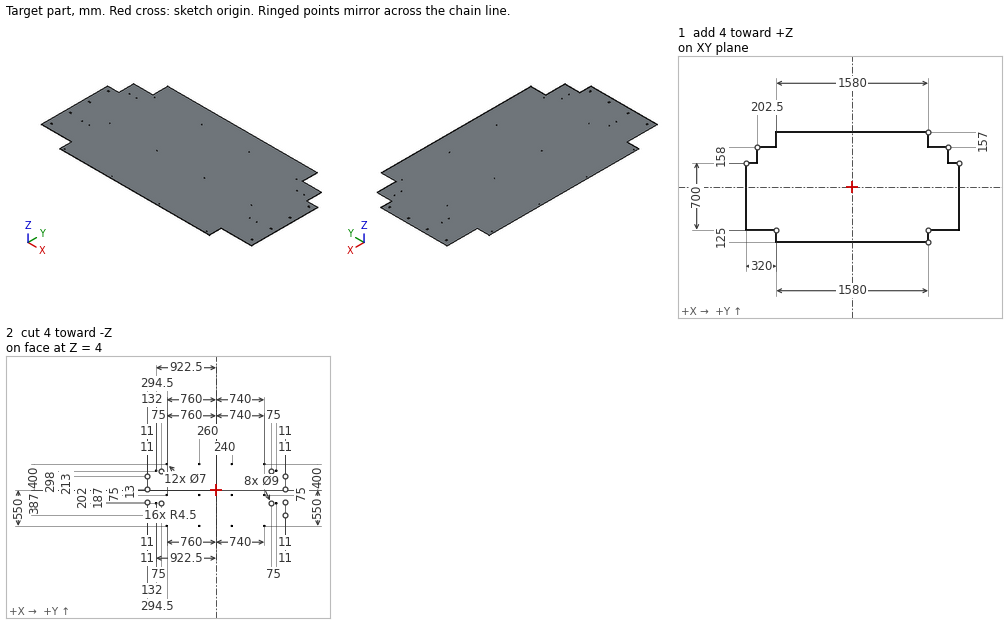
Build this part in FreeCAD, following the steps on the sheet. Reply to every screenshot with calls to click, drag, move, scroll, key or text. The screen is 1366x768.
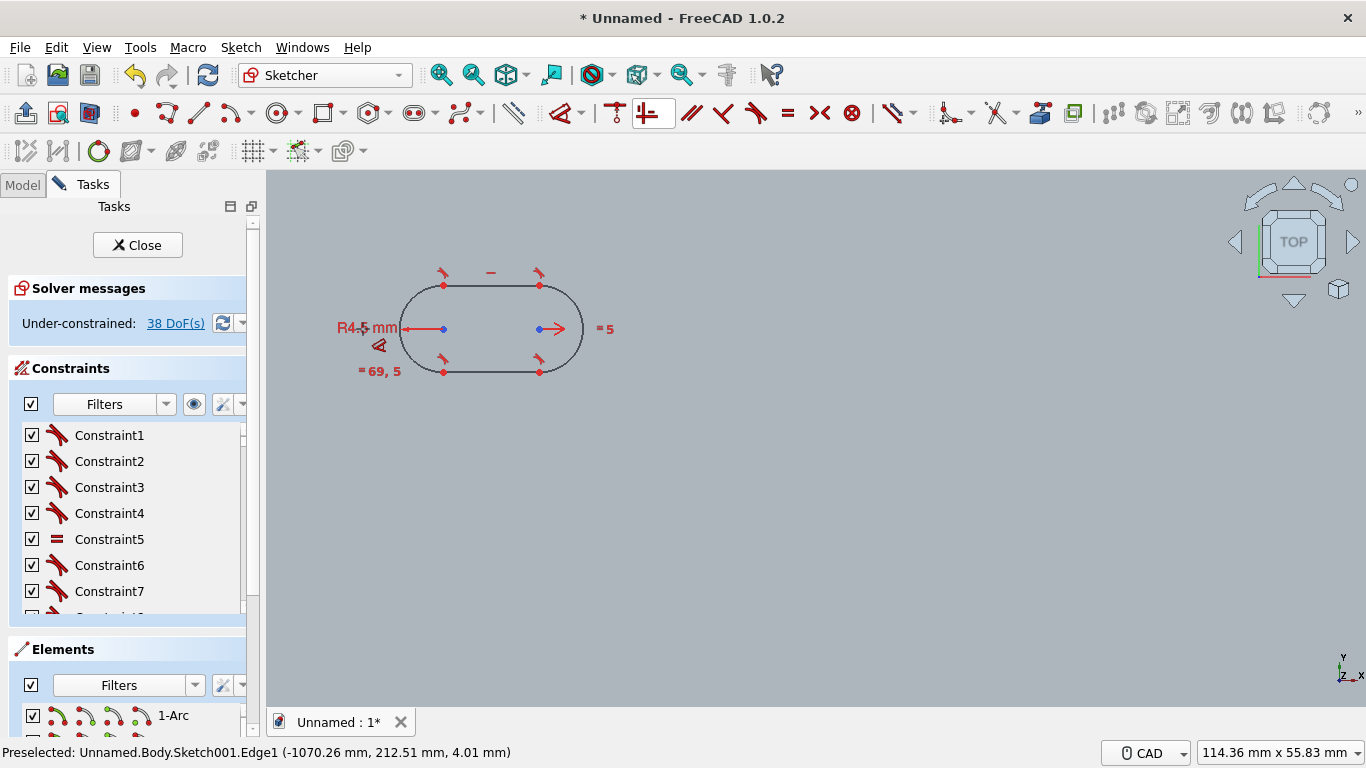
click(472, 286)
click(491, 252)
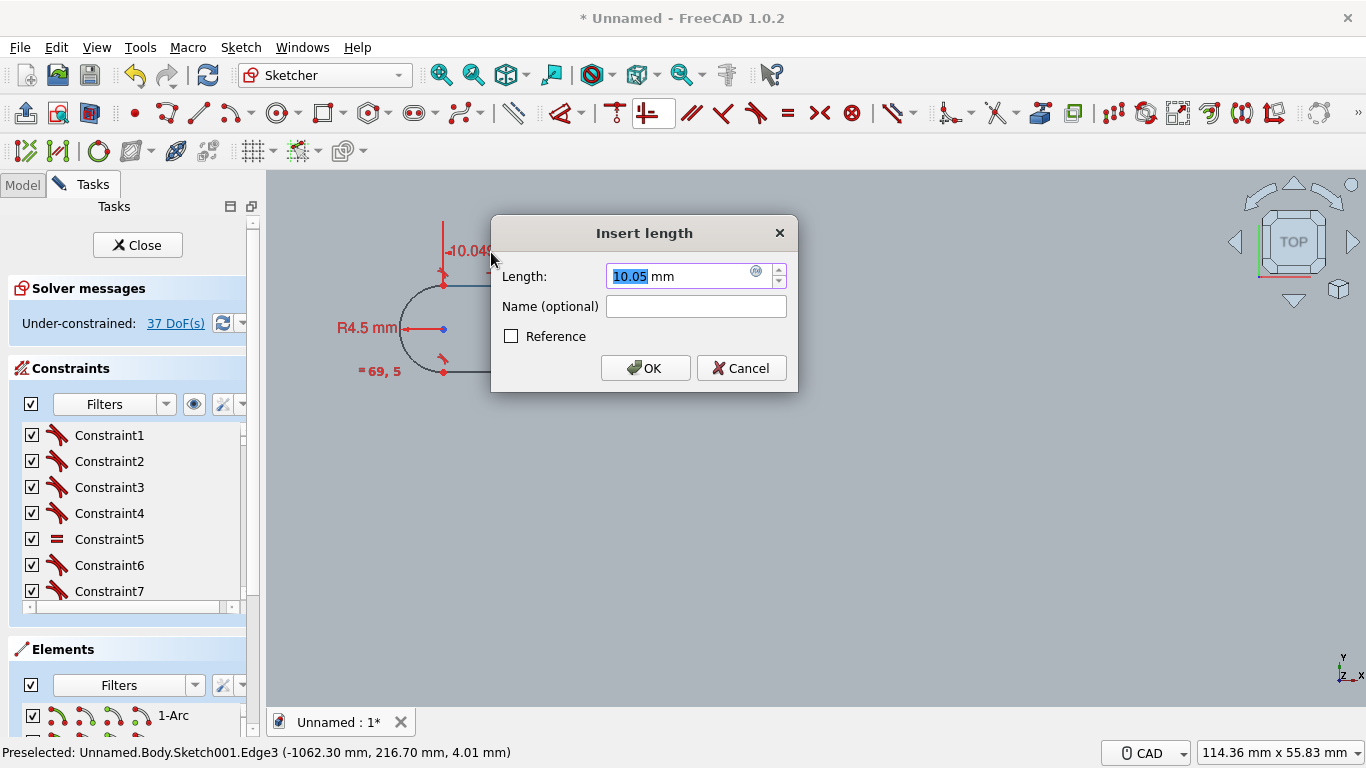
text(11)
key(Return)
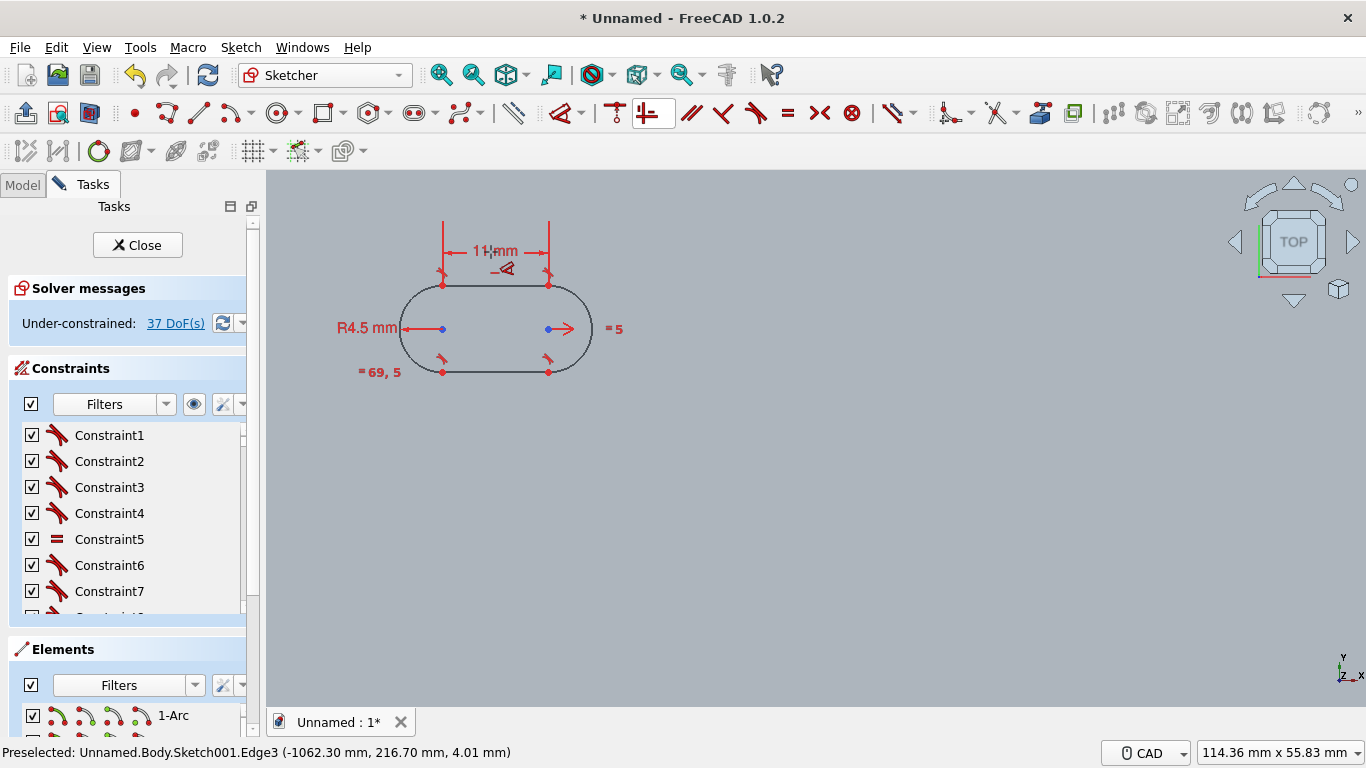
scroll(325, 326, down, 16)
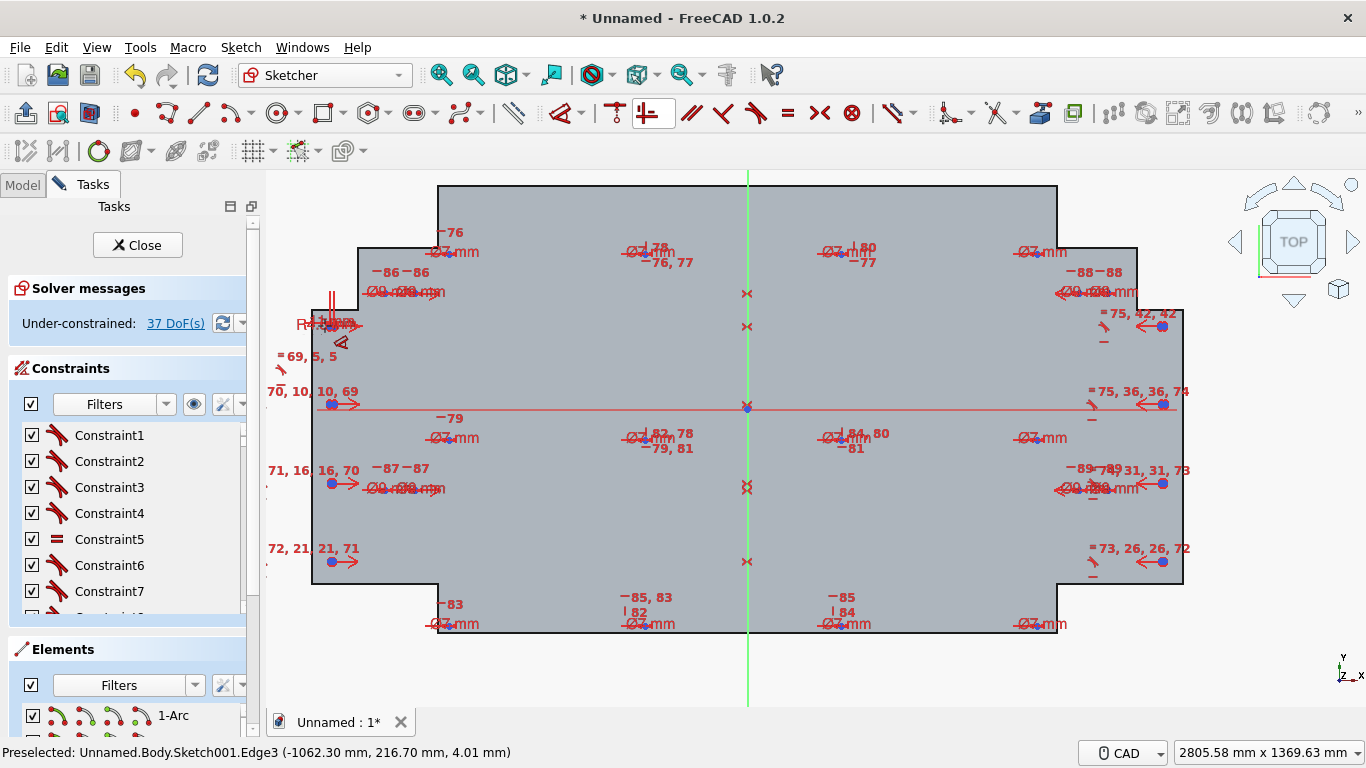
scroll(331, 403, up, 13)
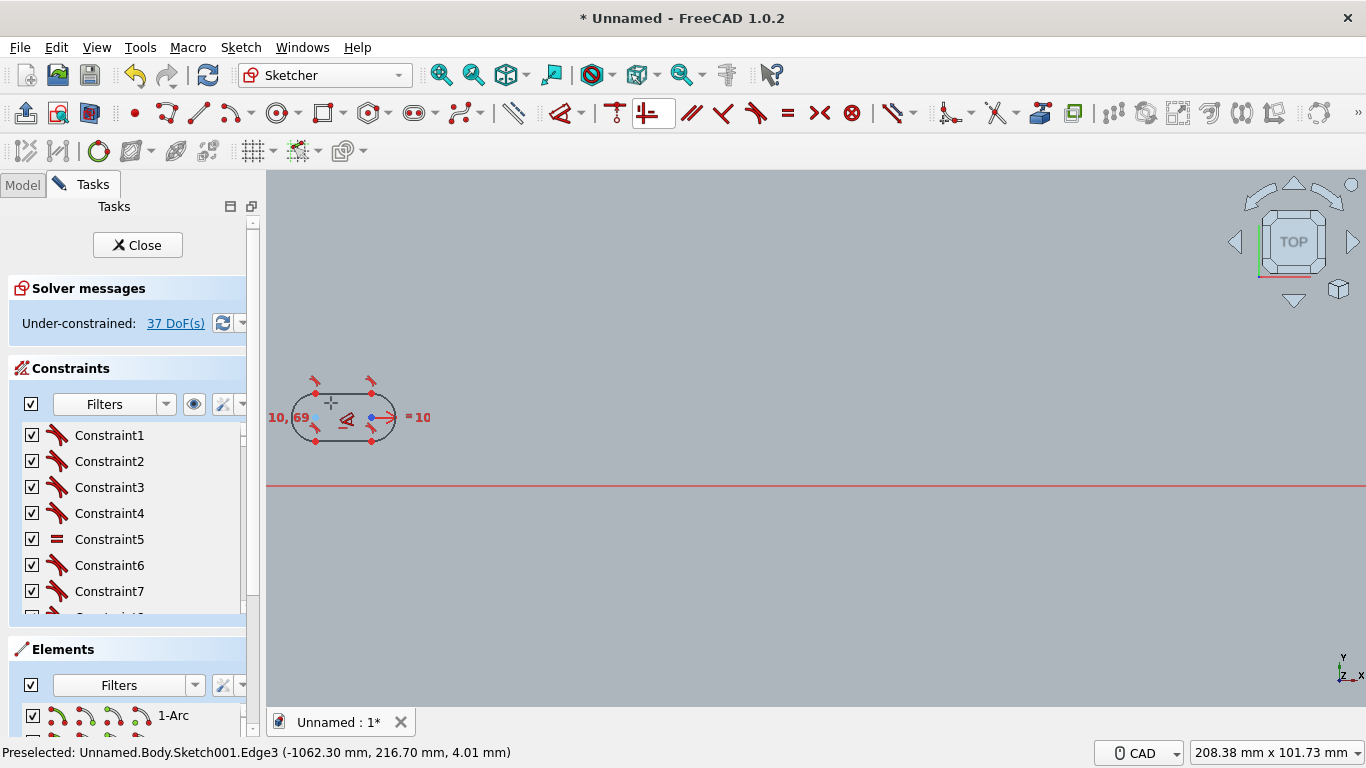
click(332, 394)
click(344, 360)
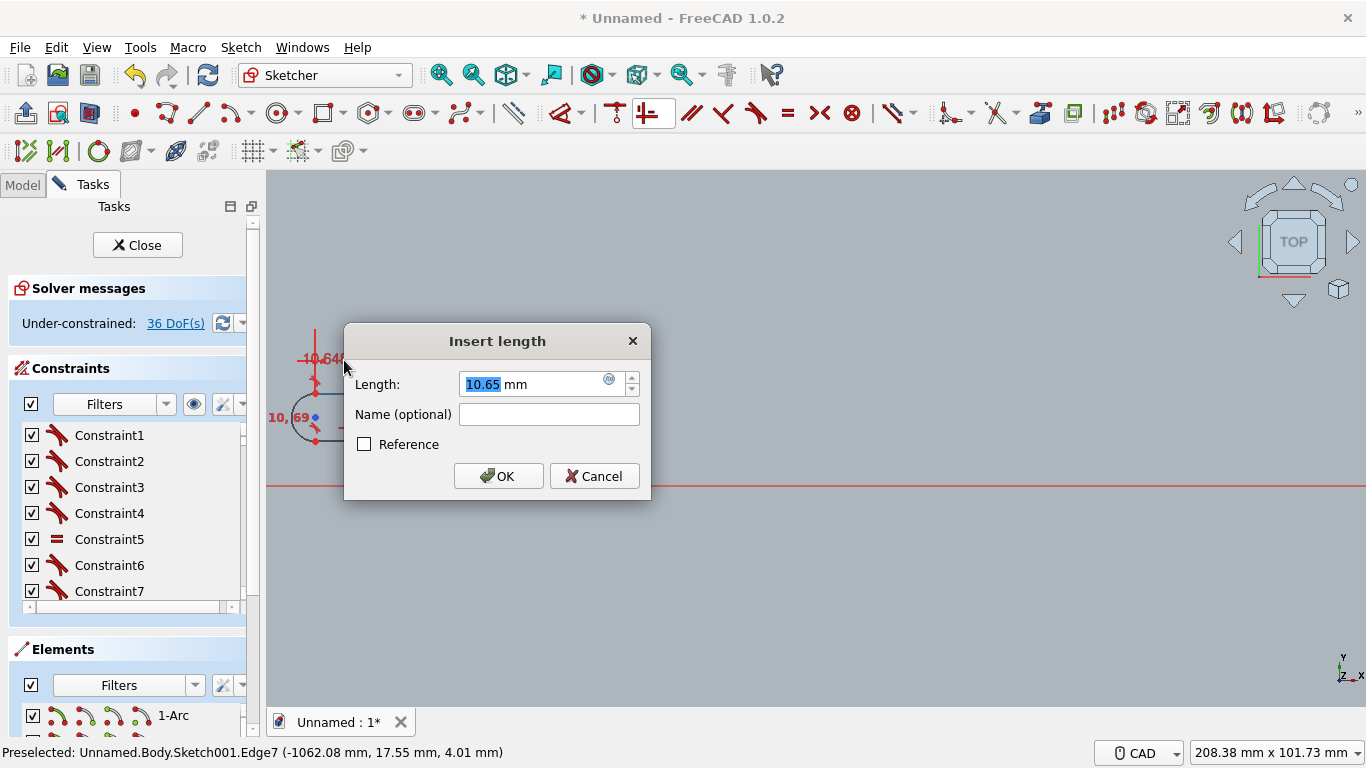
text(11)
key(Return)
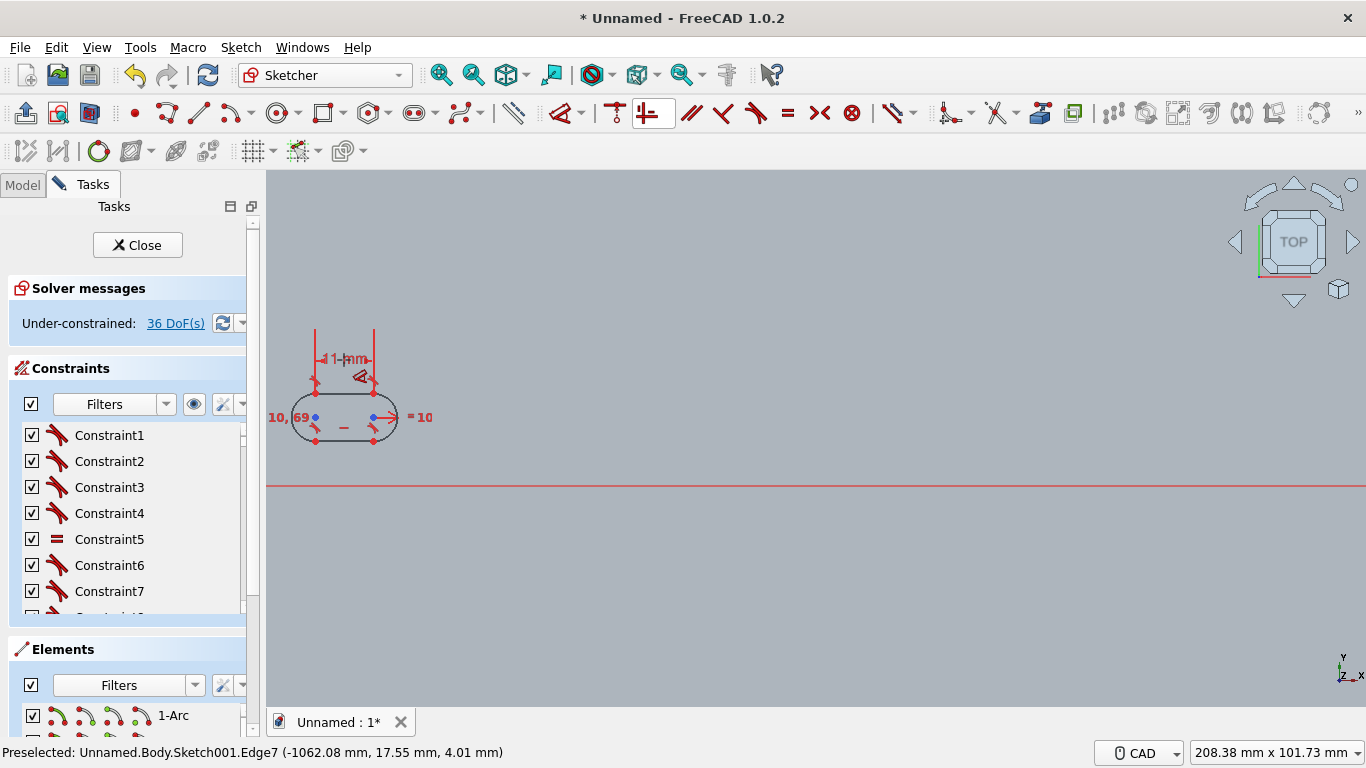
scroll(411, 410, down, 14)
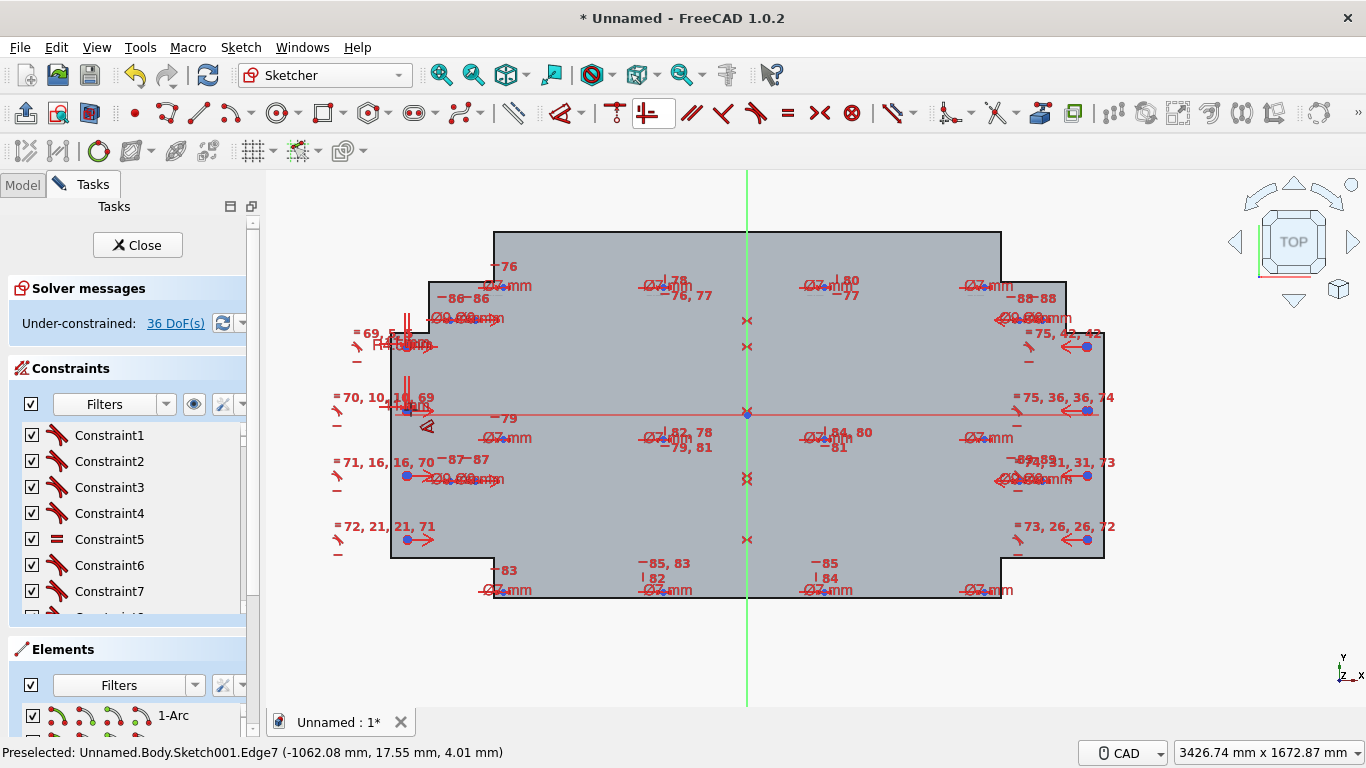
scroll(406, 474, up, 14)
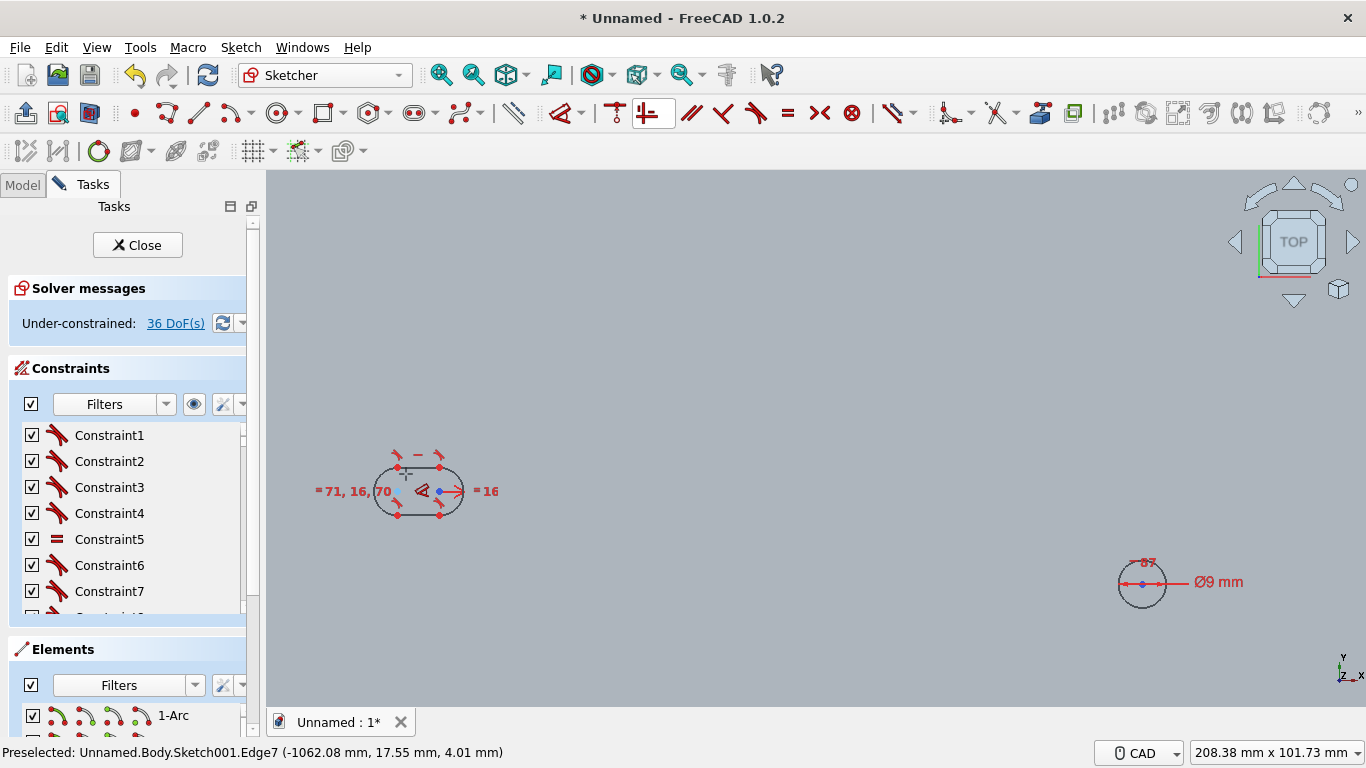
click(410, 468)
click(419, 502)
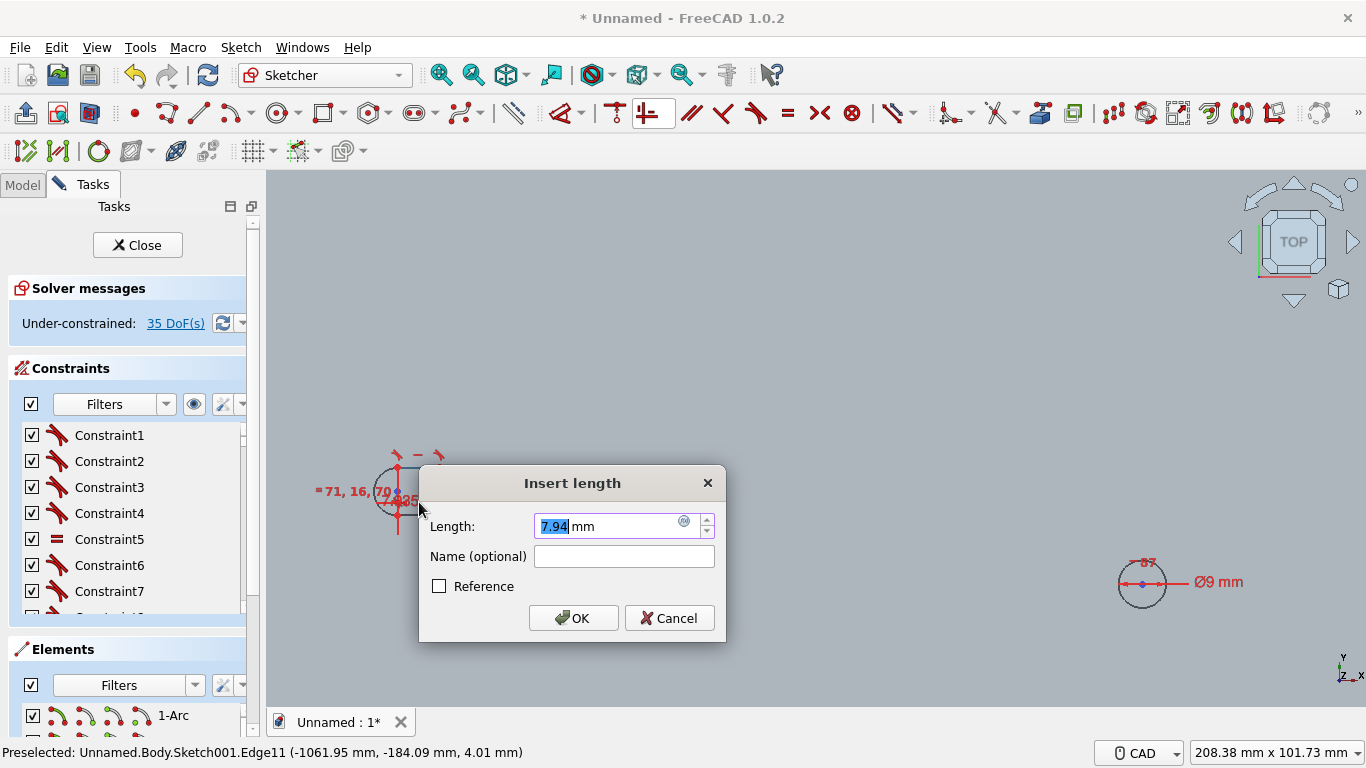
text(11)
key(Return)